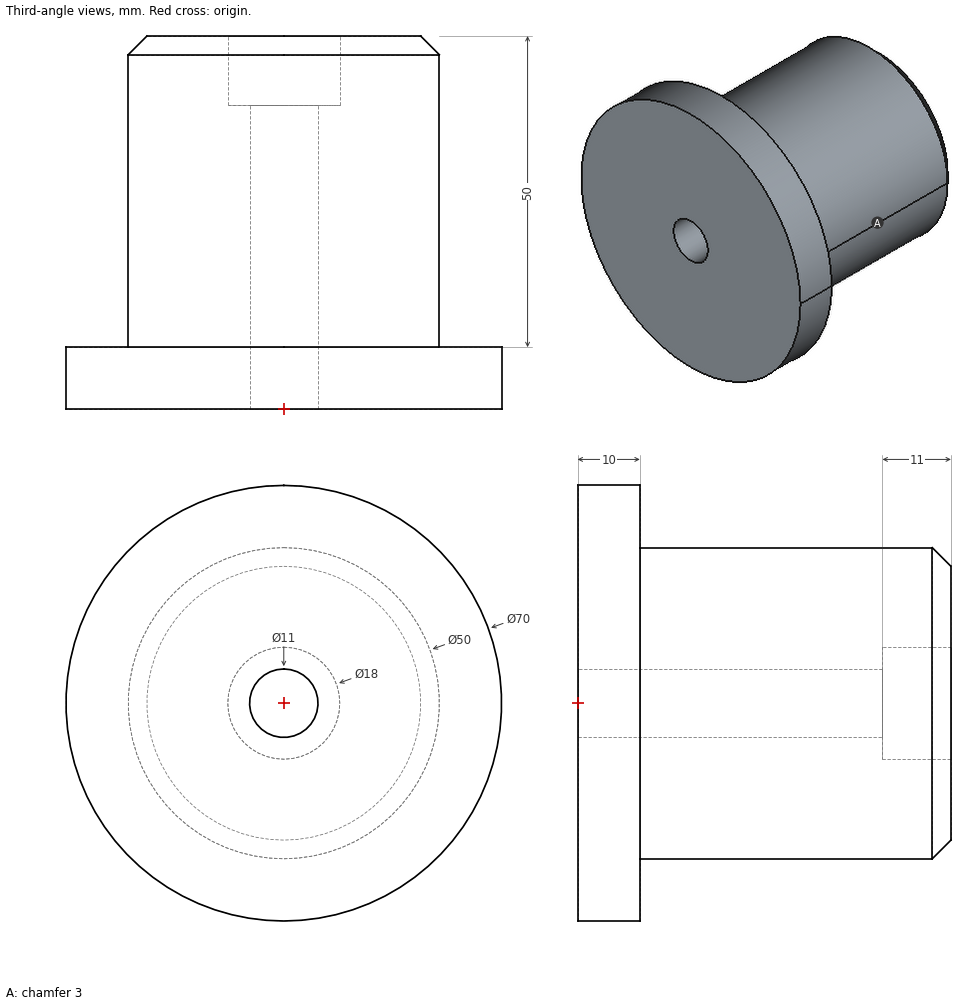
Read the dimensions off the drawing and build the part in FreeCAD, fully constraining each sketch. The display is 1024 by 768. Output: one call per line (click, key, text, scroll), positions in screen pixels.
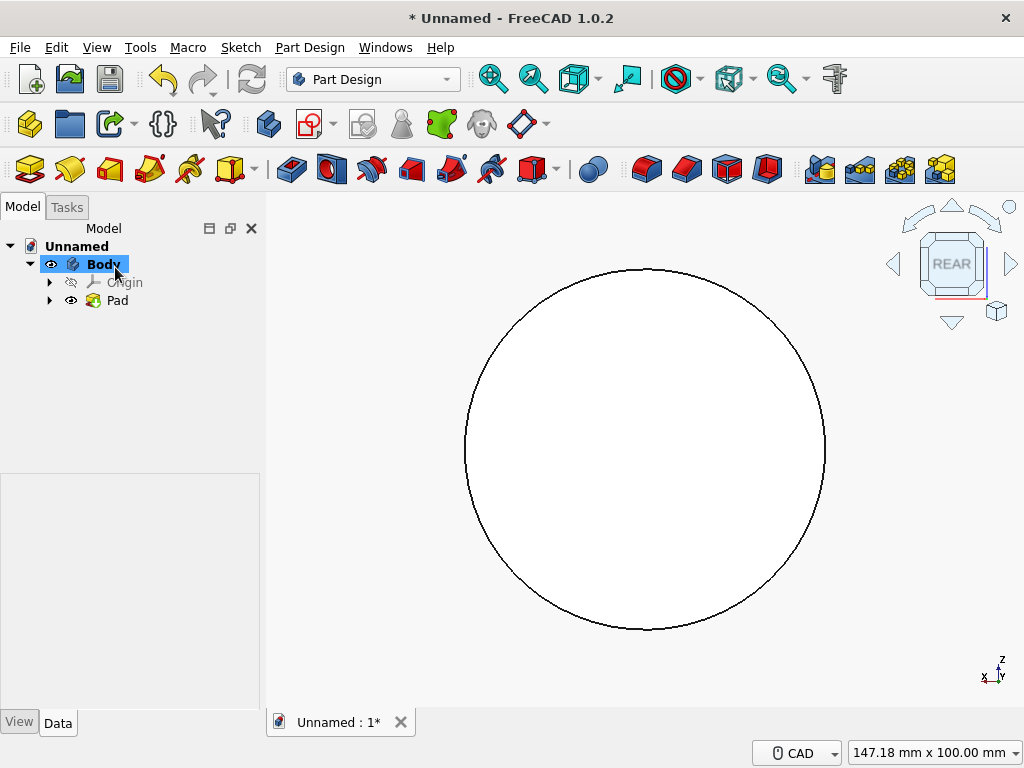
click(645, 448)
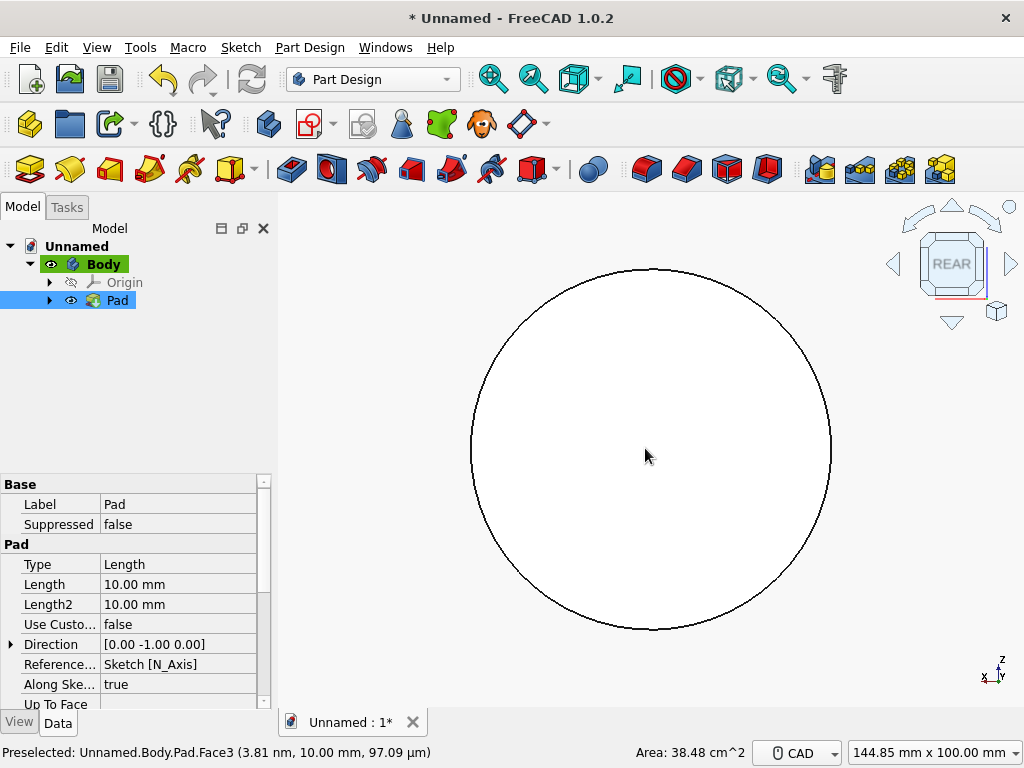
click(310, 124)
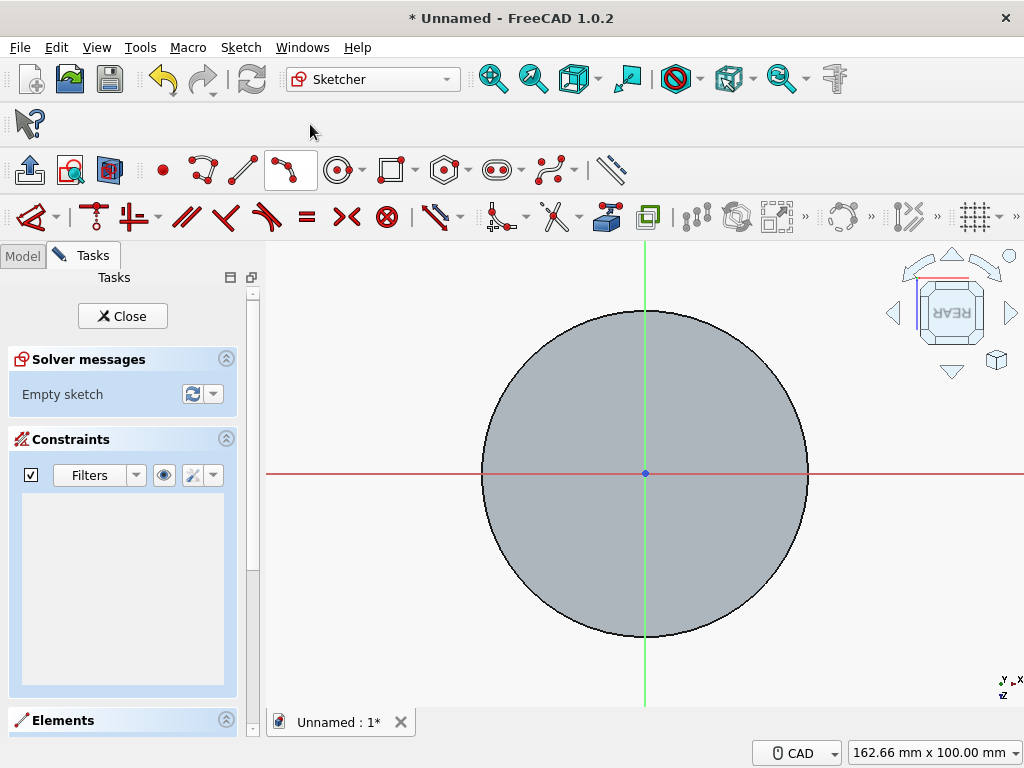
click(338, 170)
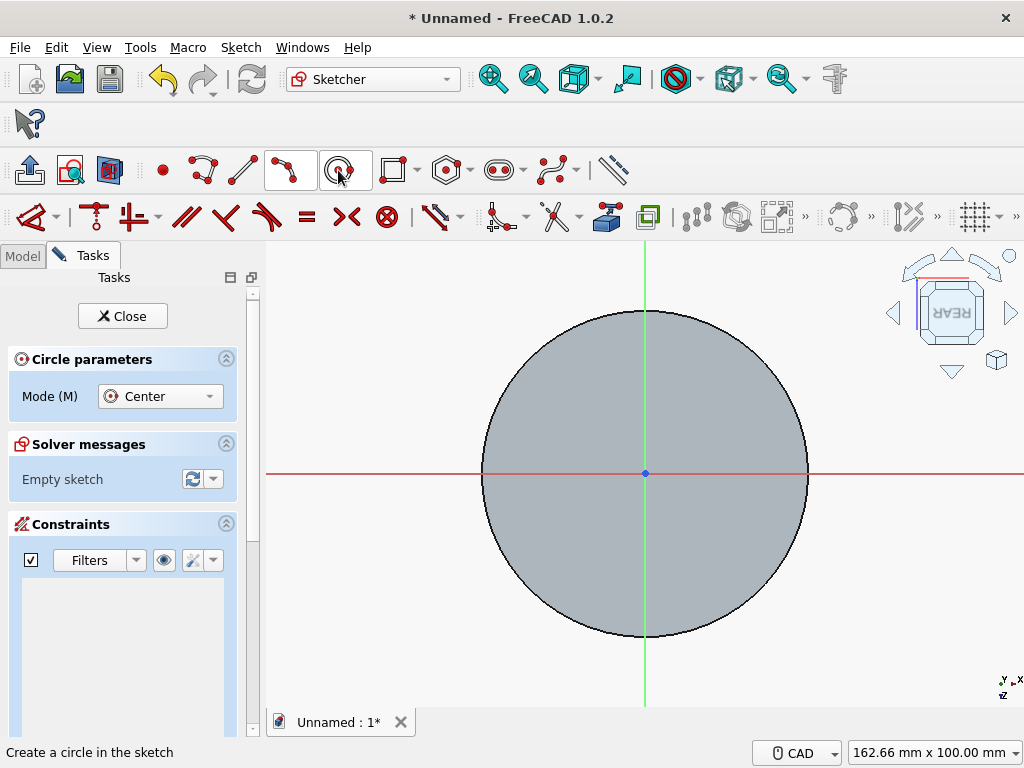
click(645, 474)
move(727, 392)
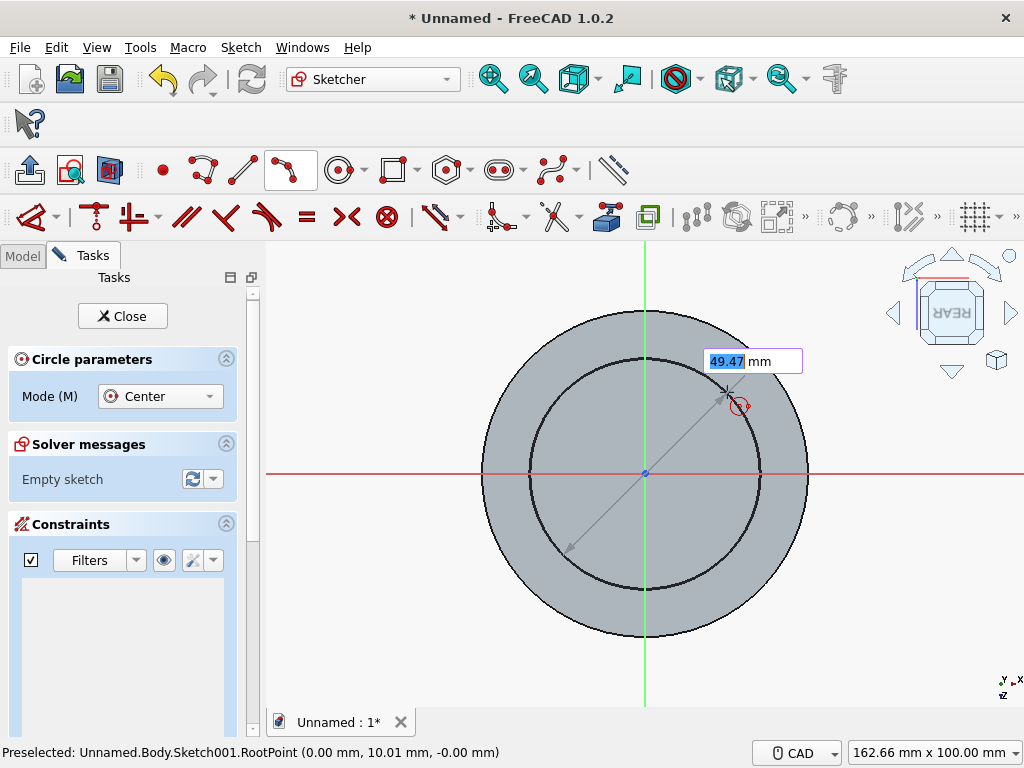
text(50)
key(Return)
key(Escape)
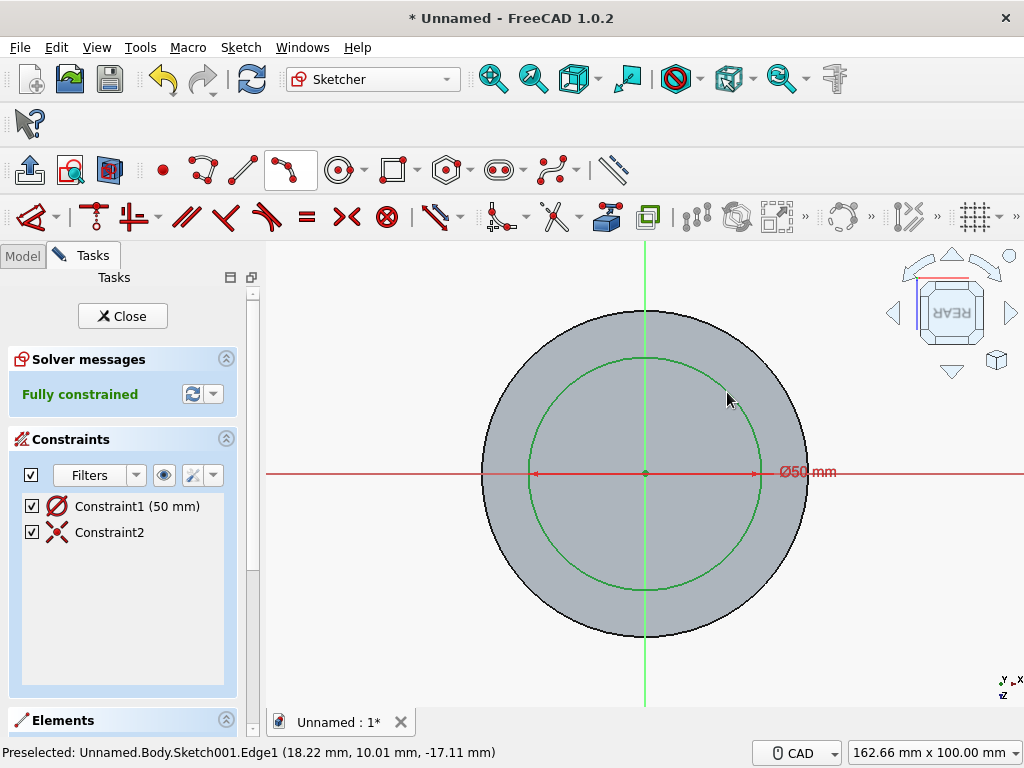
click(123, 316)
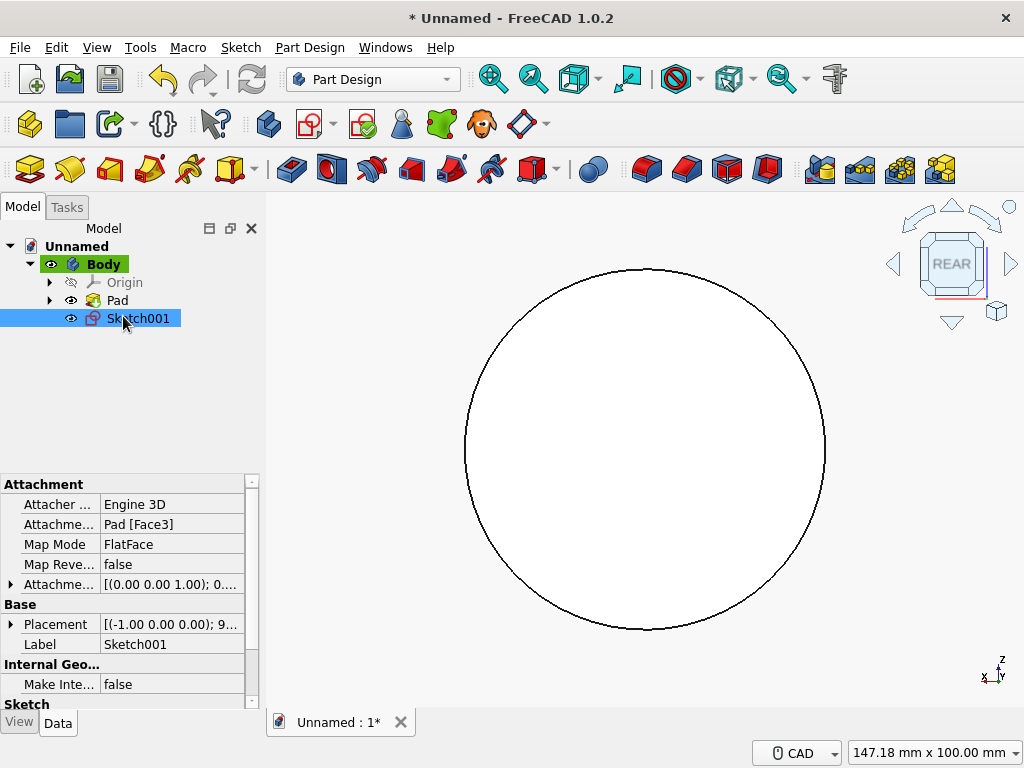
click(30, 170)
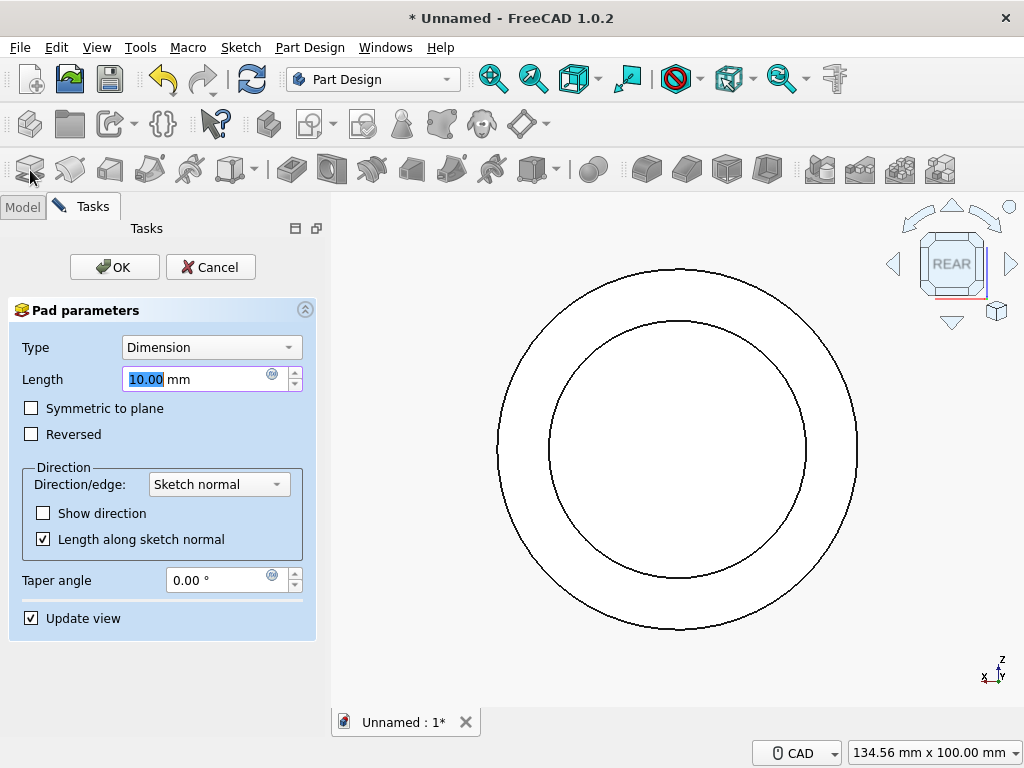
text(50)
key(Tab)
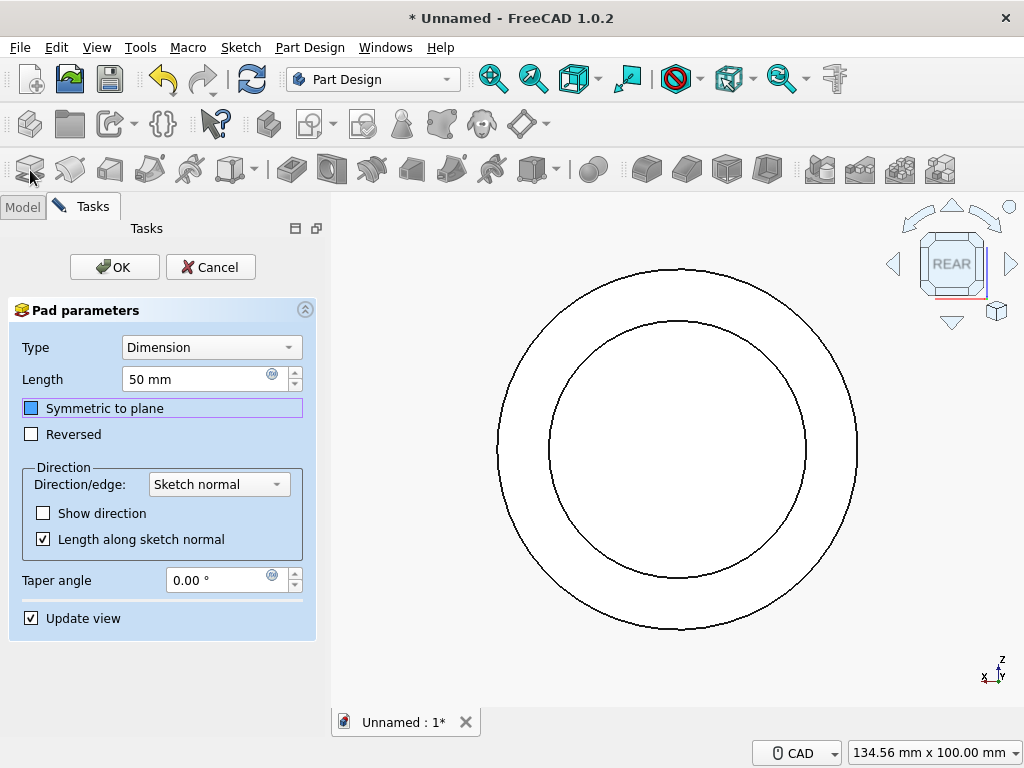
click(115, 267)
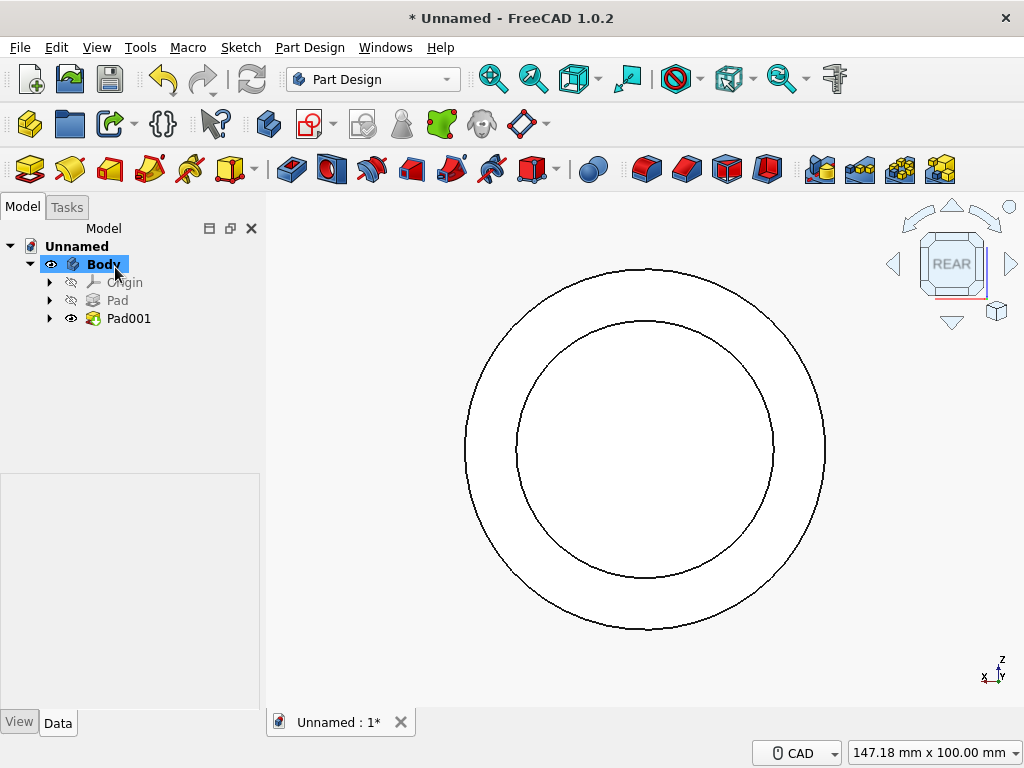
click(774, 449)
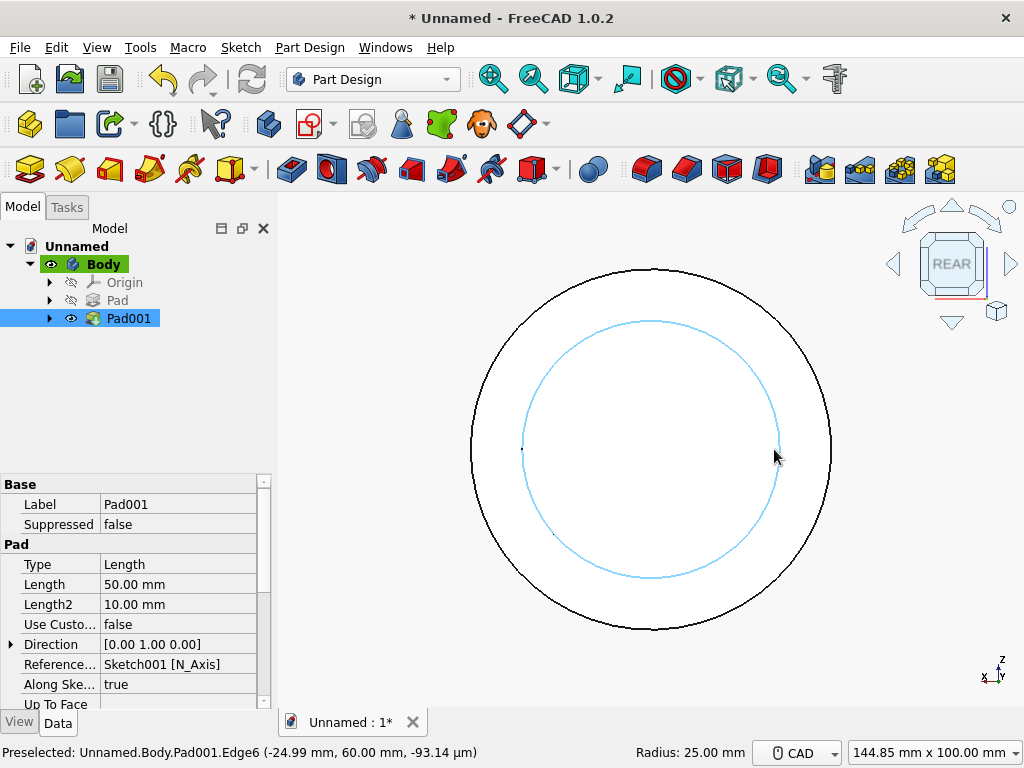
click(688, 170)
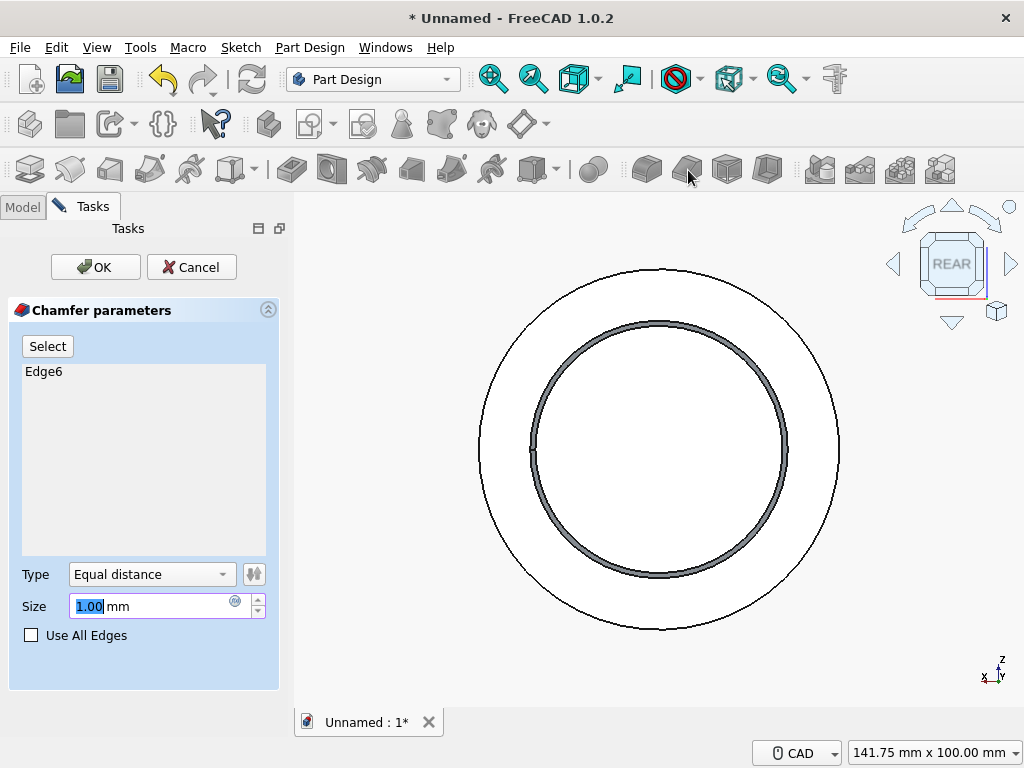
text(3)
key(Tab)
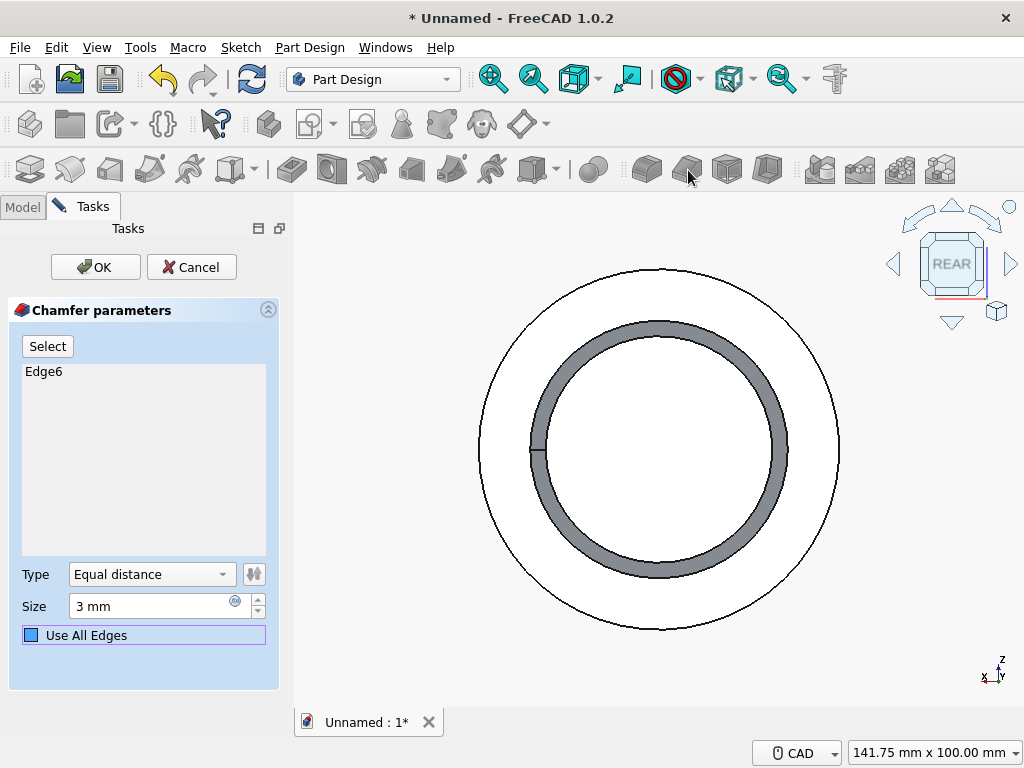
click(96, 267)